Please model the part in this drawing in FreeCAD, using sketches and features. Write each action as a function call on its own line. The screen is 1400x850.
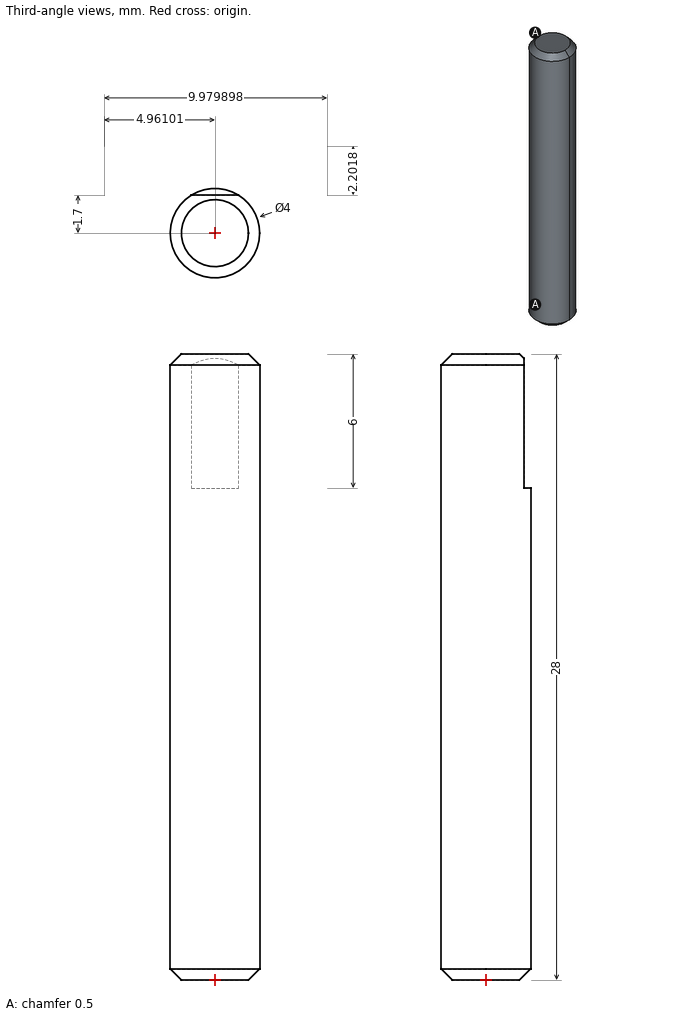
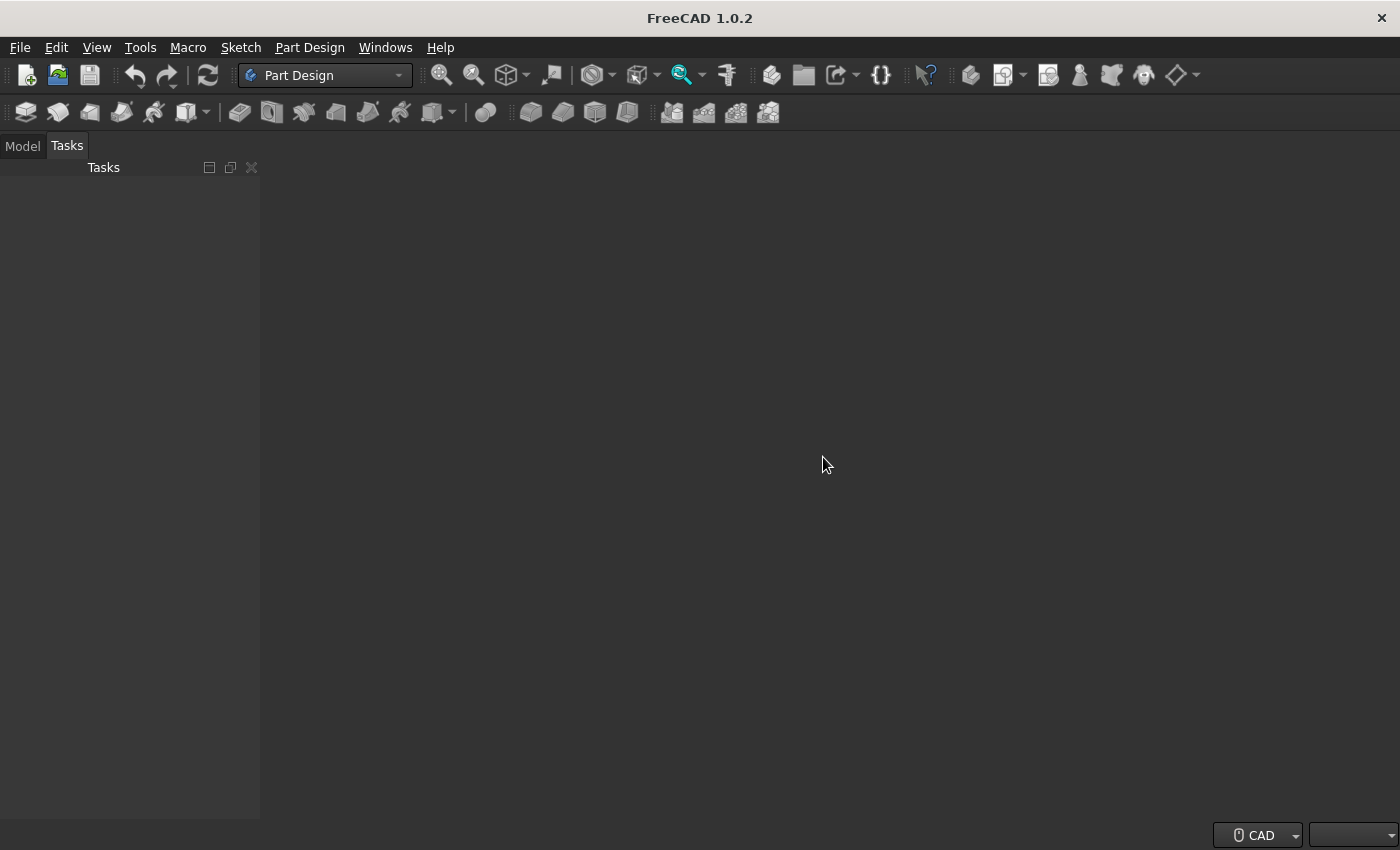
click(26, 76)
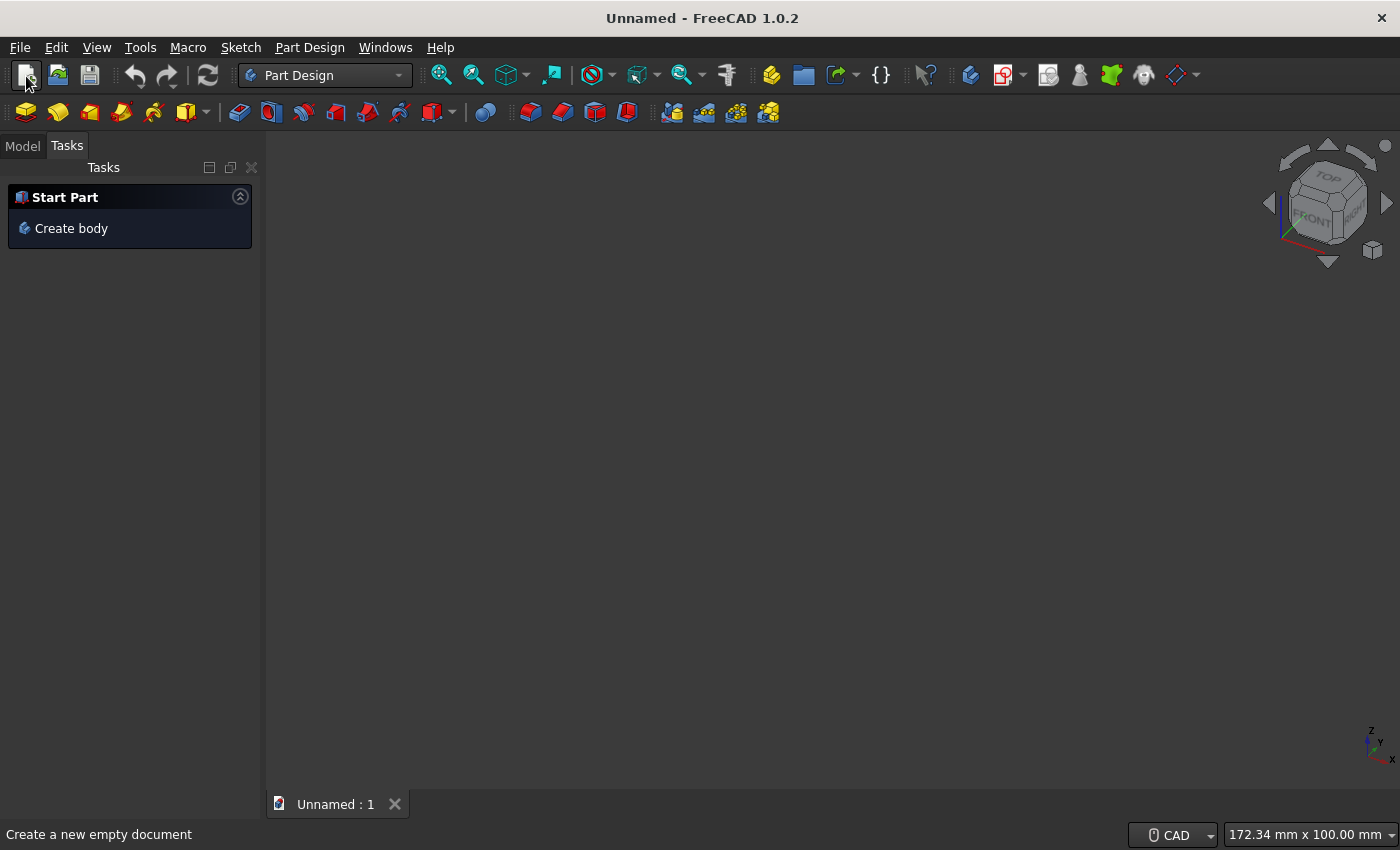
click(1004, 76)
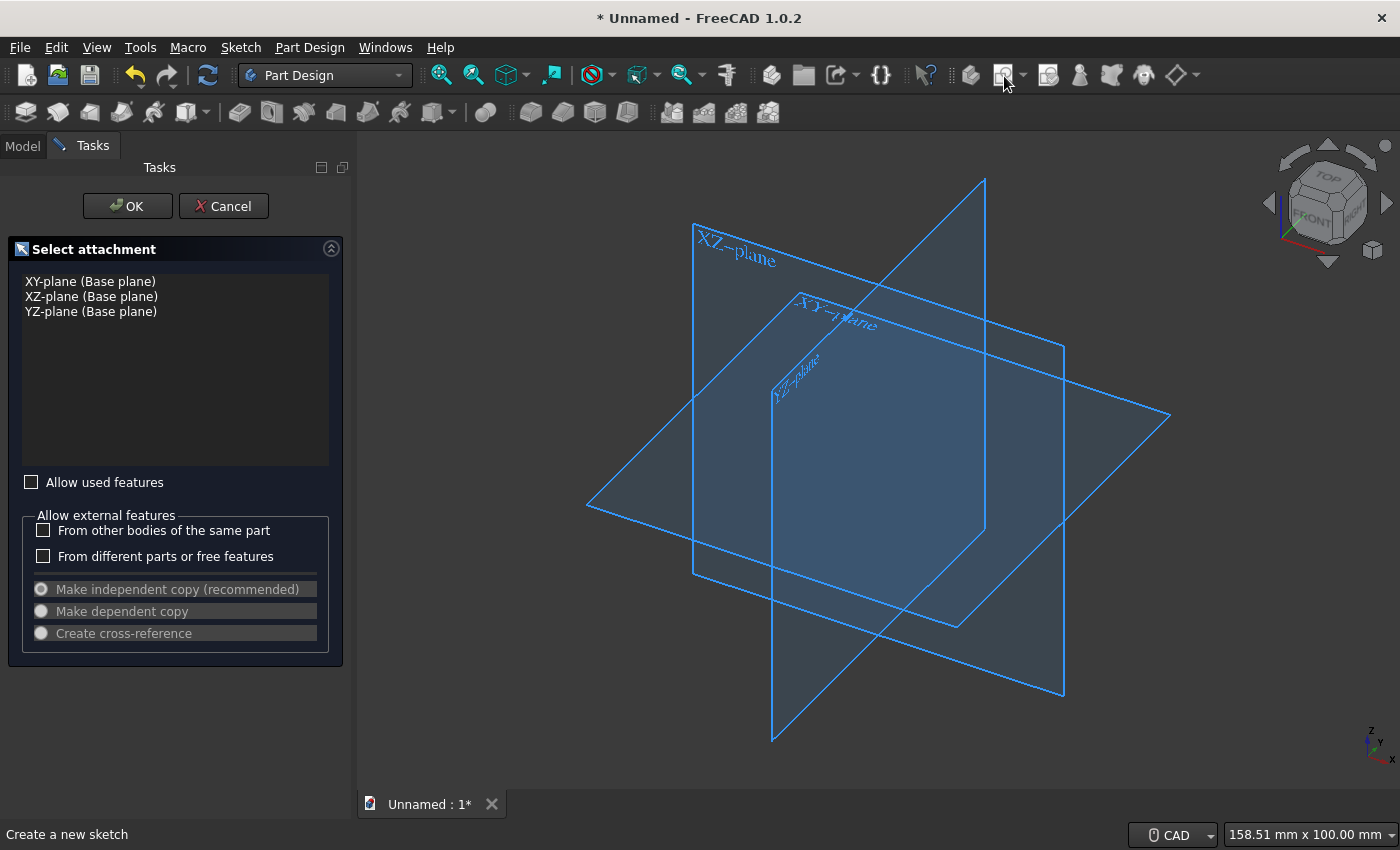
click(82, 282)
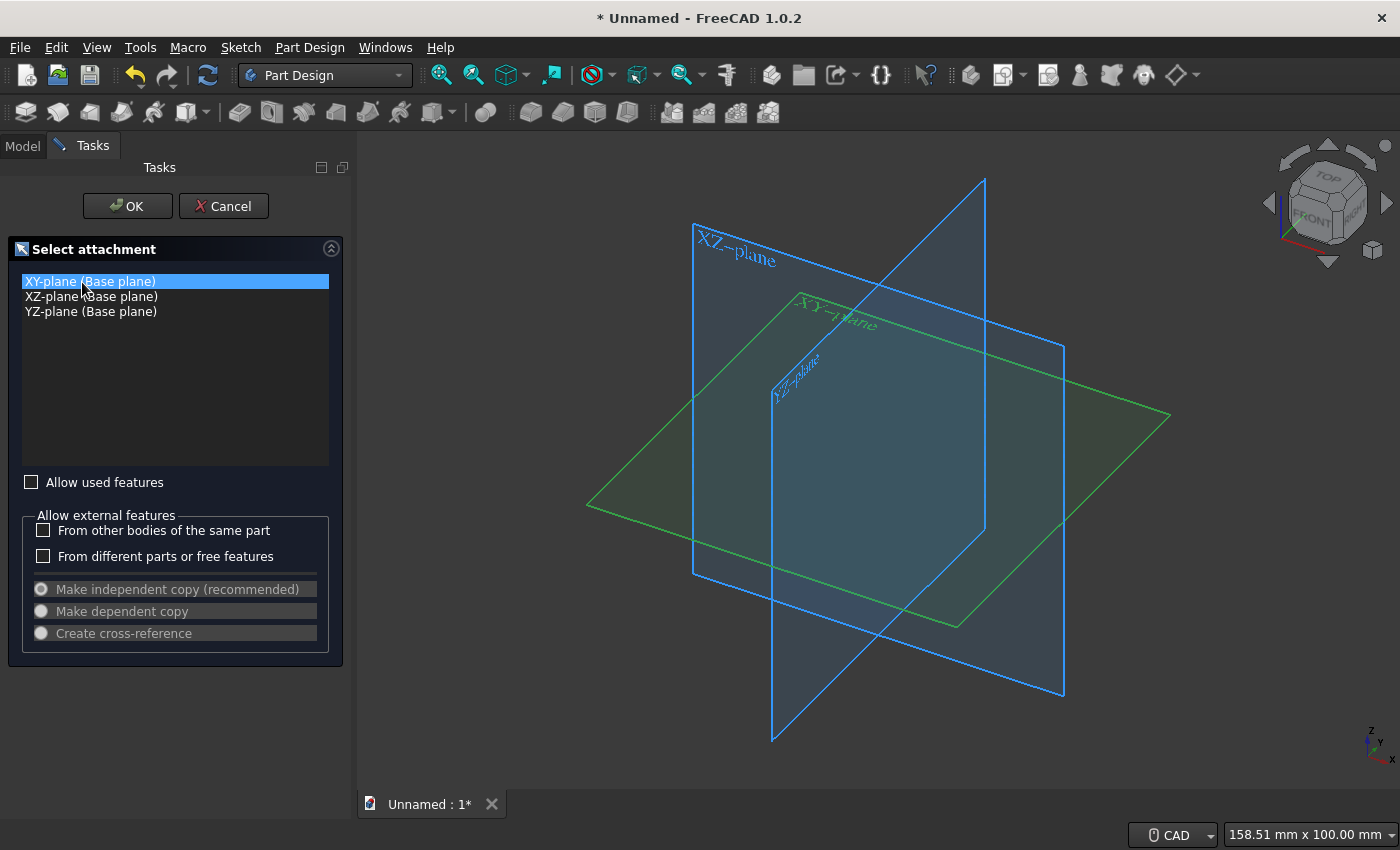
click(128, 206)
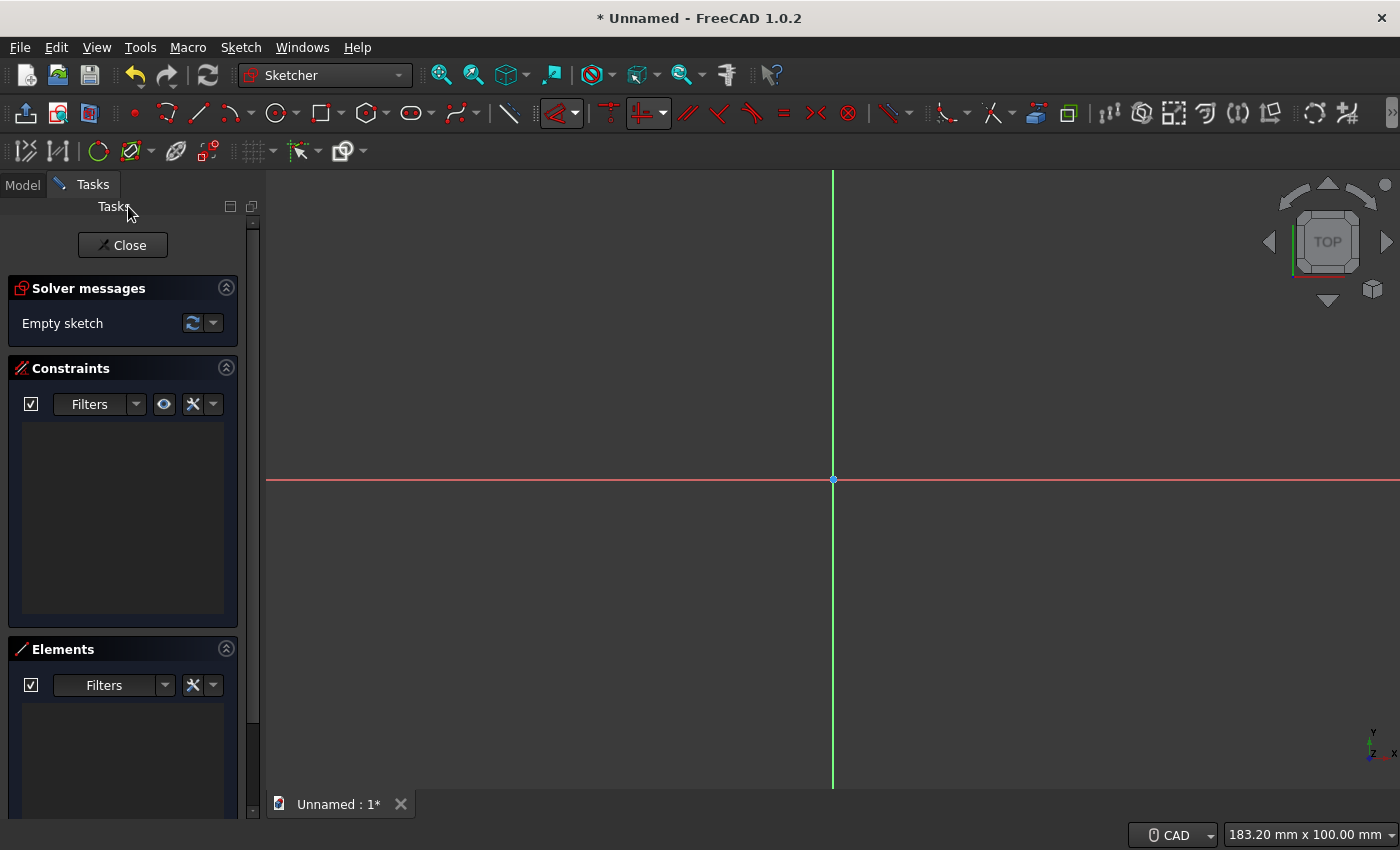
scroll(837, 480, up, 14)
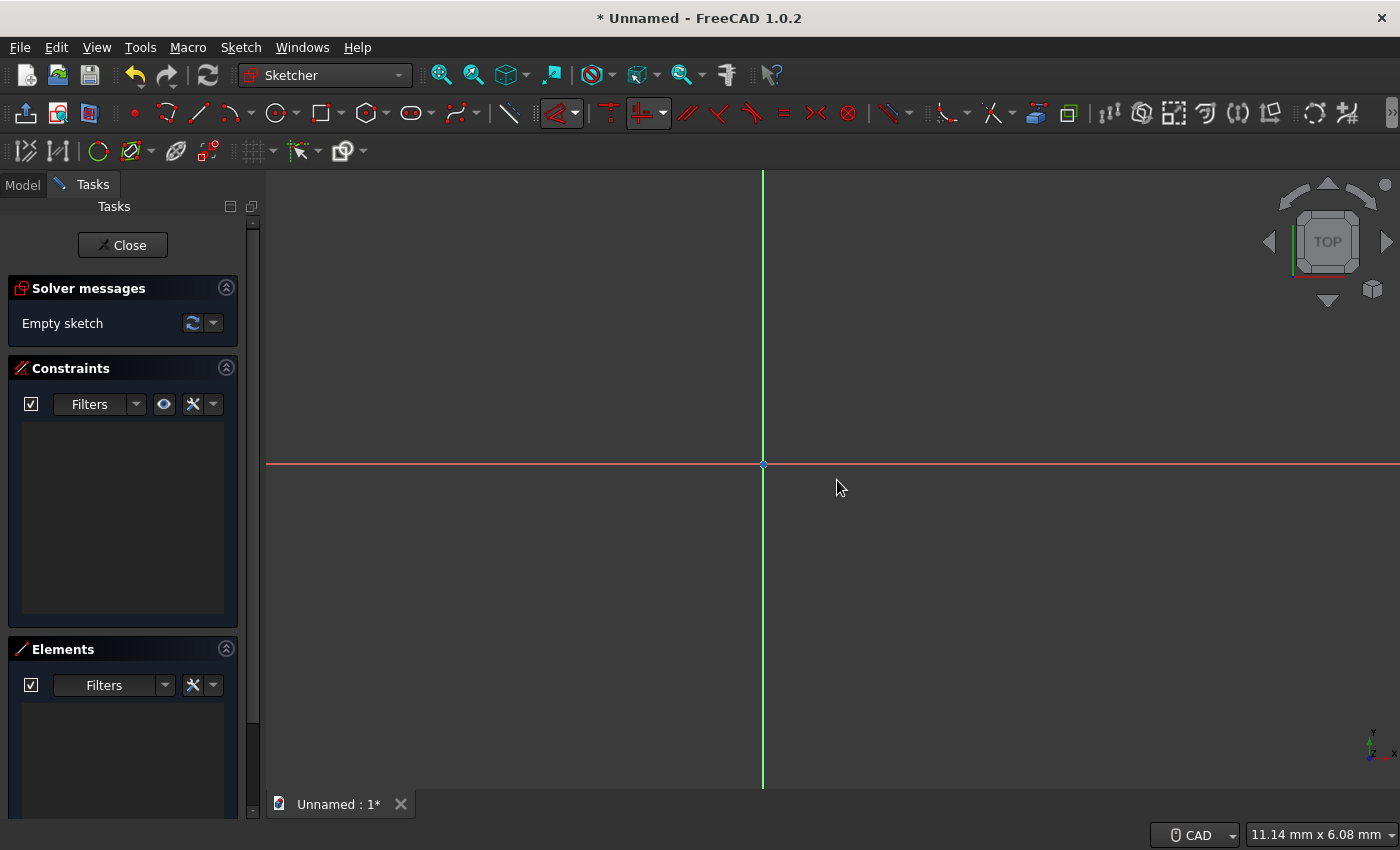
click(276, 114)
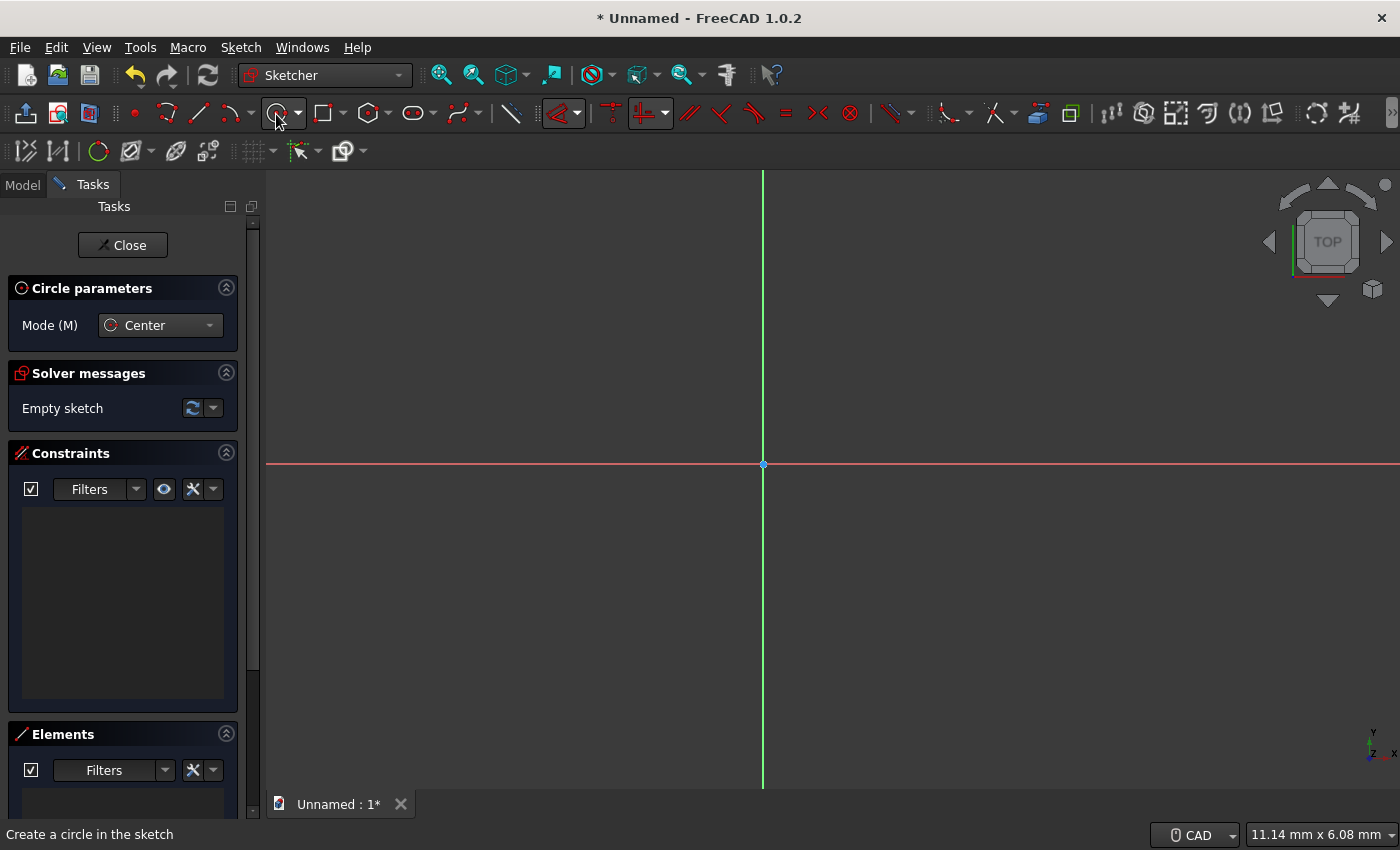
click(763, 464)
move(907, 320)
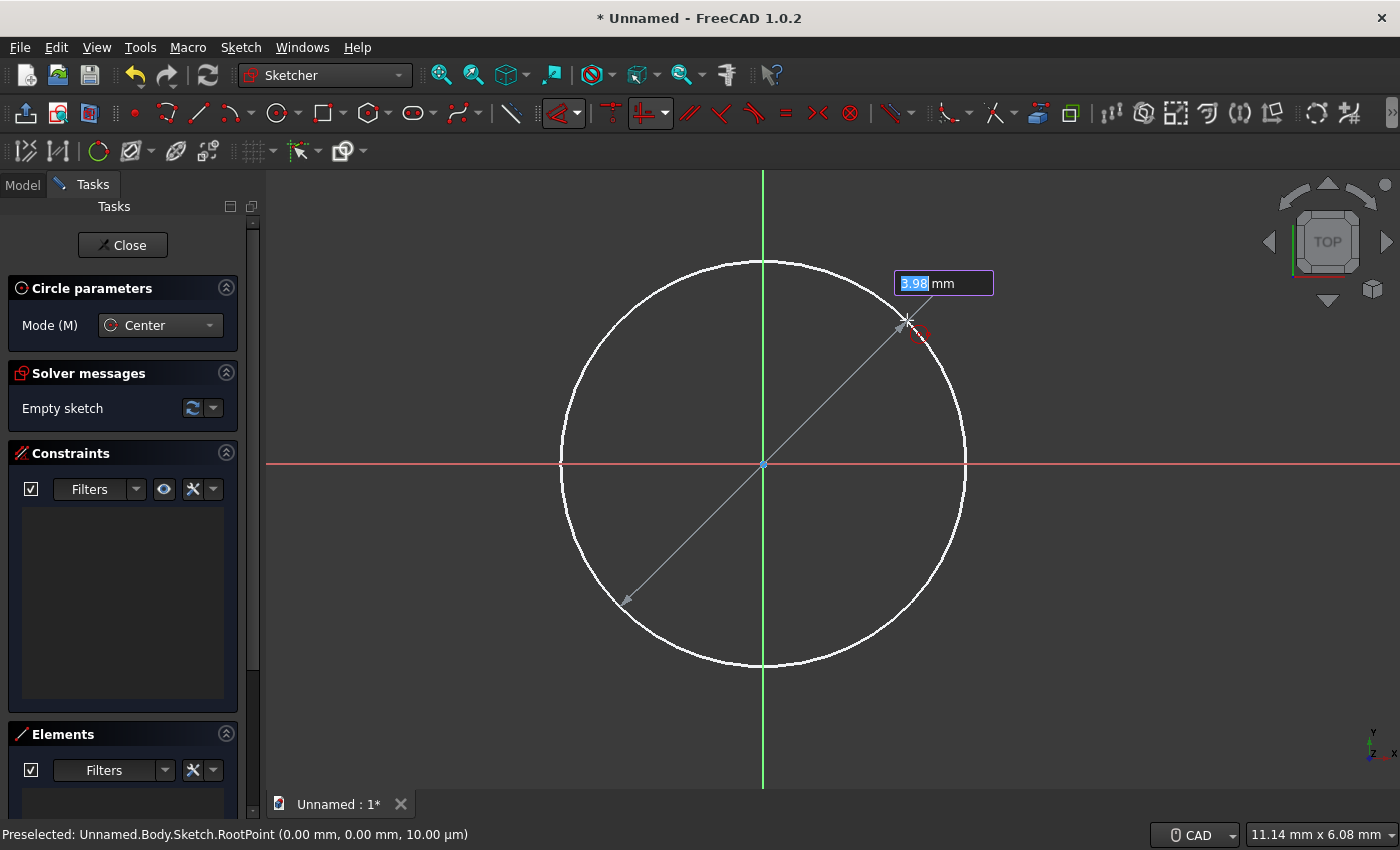
text(4)
key(Return)
key(Escape)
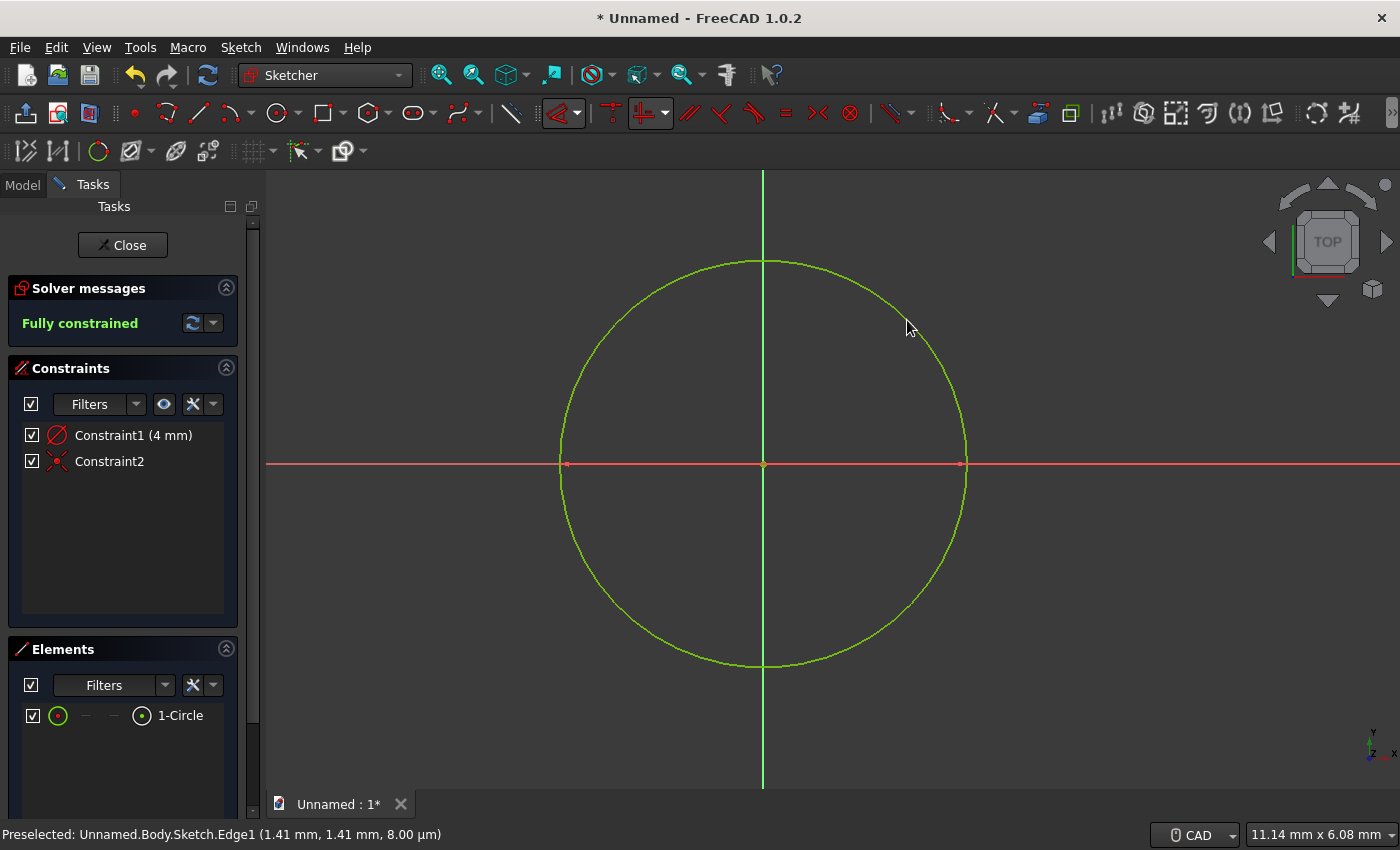
click(123, 245)